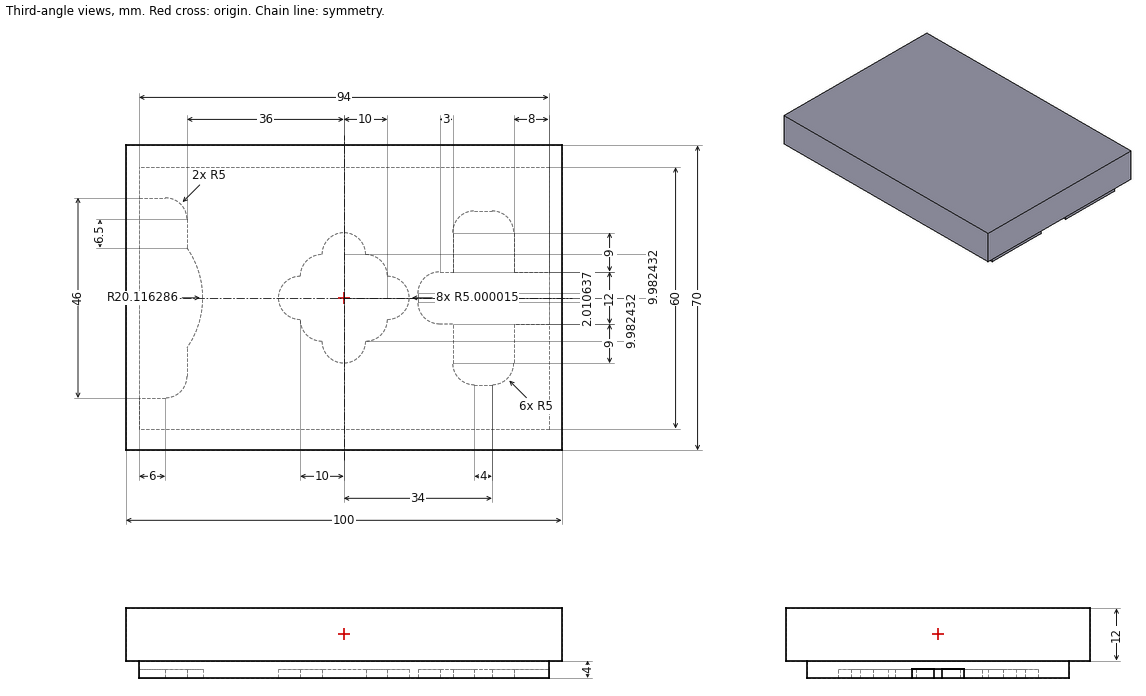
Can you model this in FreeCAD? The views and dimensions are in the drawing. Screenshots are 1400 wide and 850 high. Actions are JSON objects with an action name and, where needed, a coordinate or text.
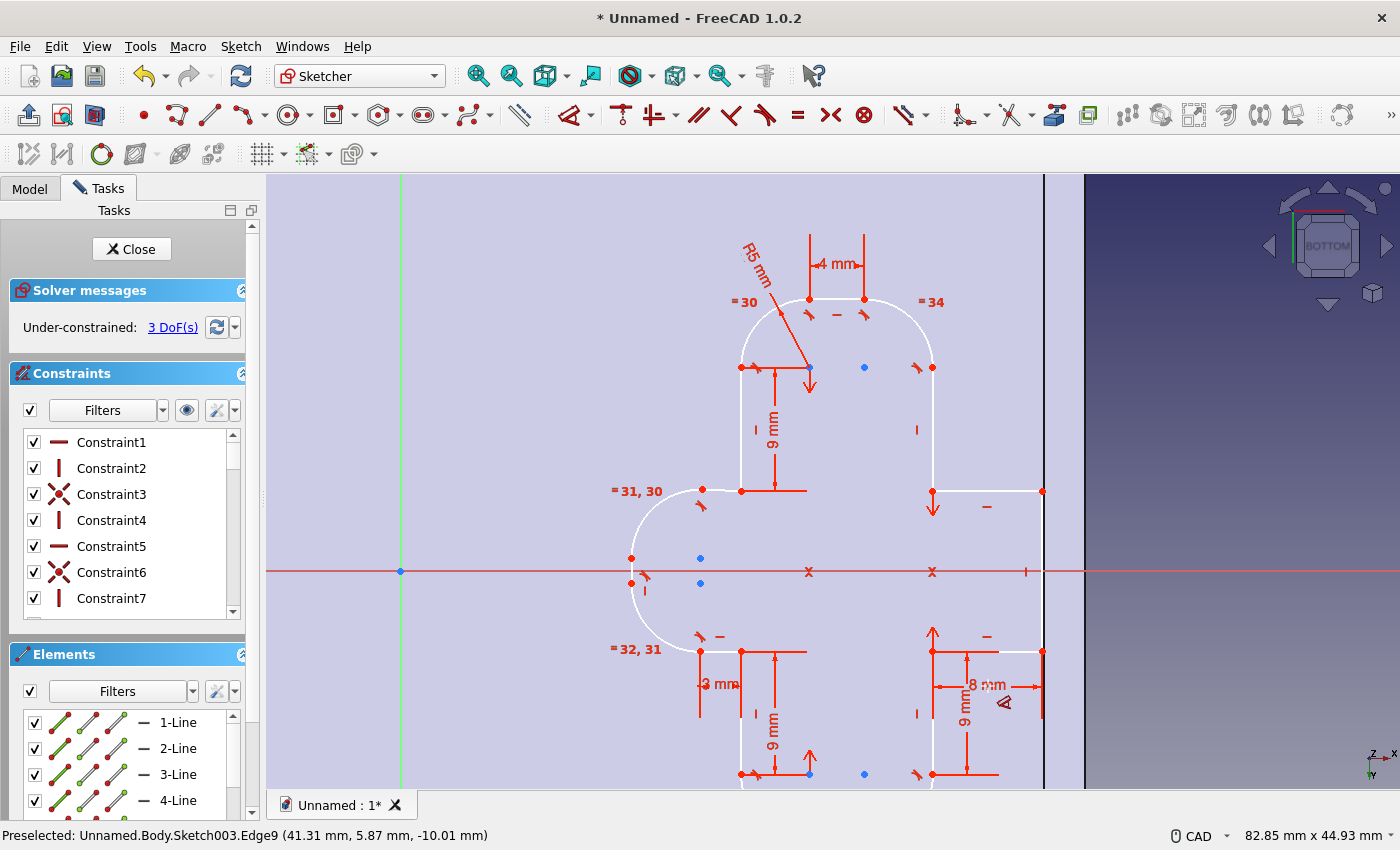
{"action": "left_click", "coordinate": [1042, 604]}
{"action": "left_click", "coordinate": [1076, 534]}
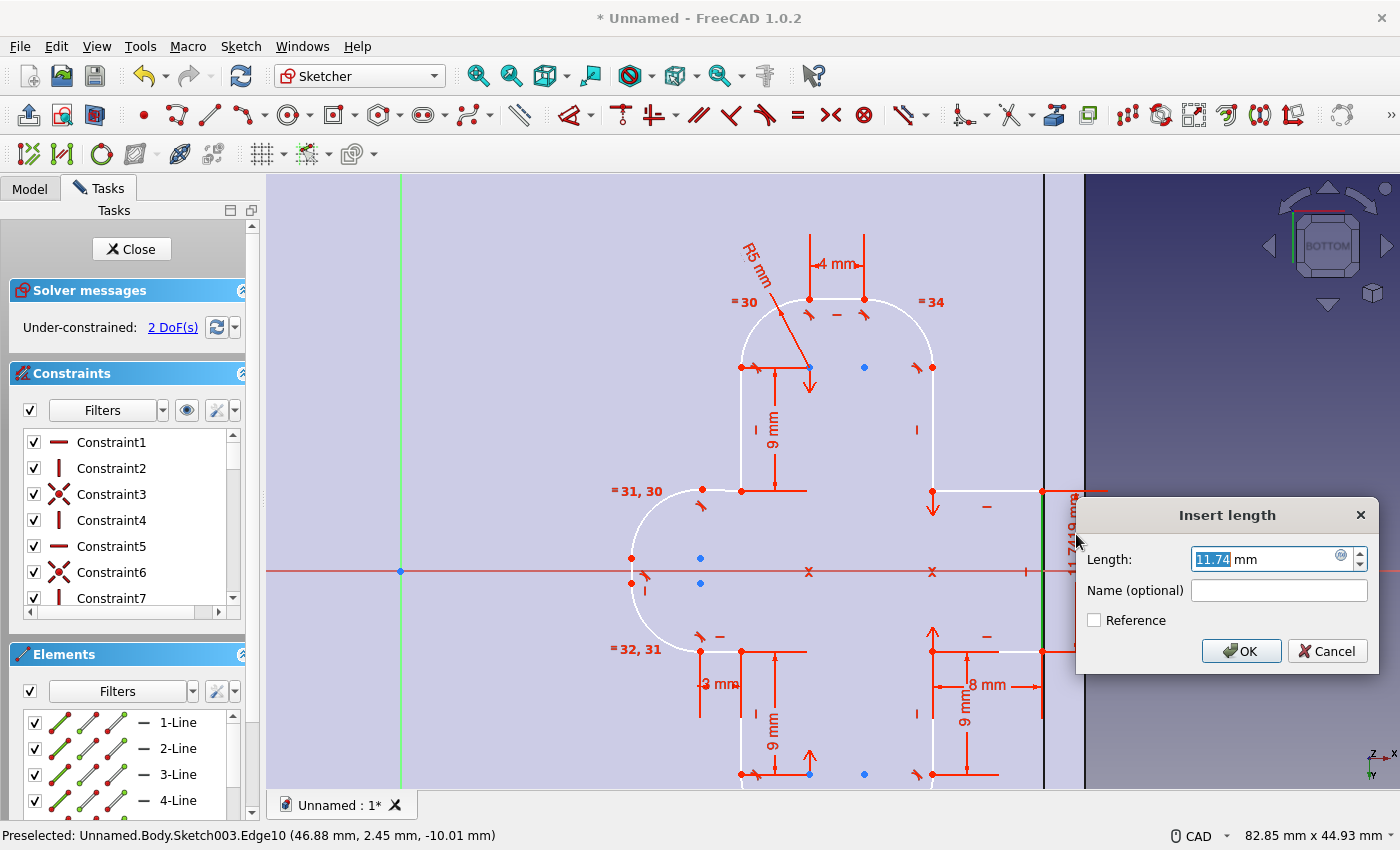
{"action": "type", "text": "12"}
{"action": "key", "text": "Return"}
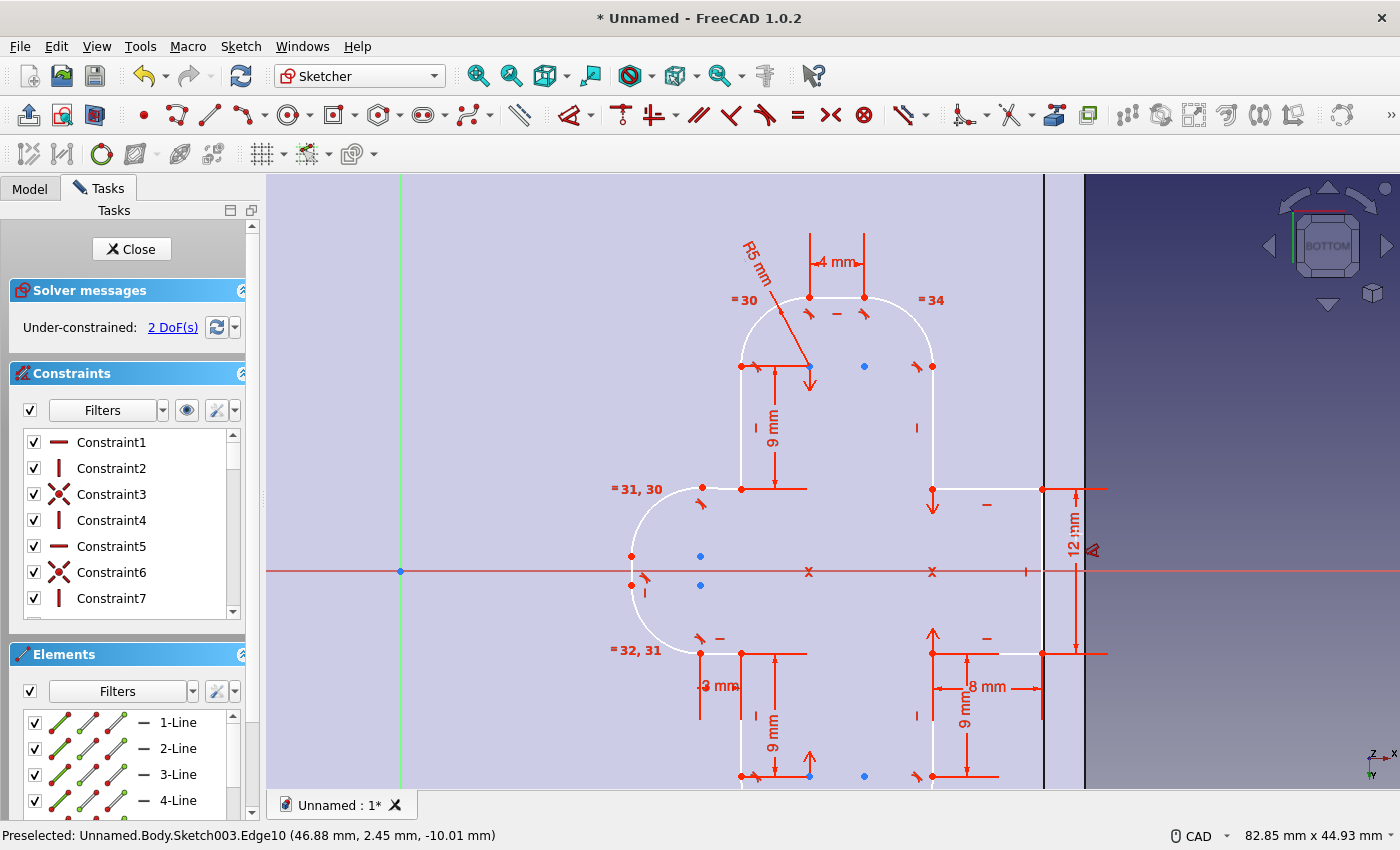
{"action": "left_click", "coordinate": [864, 298]}
{"action": "left_click", "coordinate": [633, 264]}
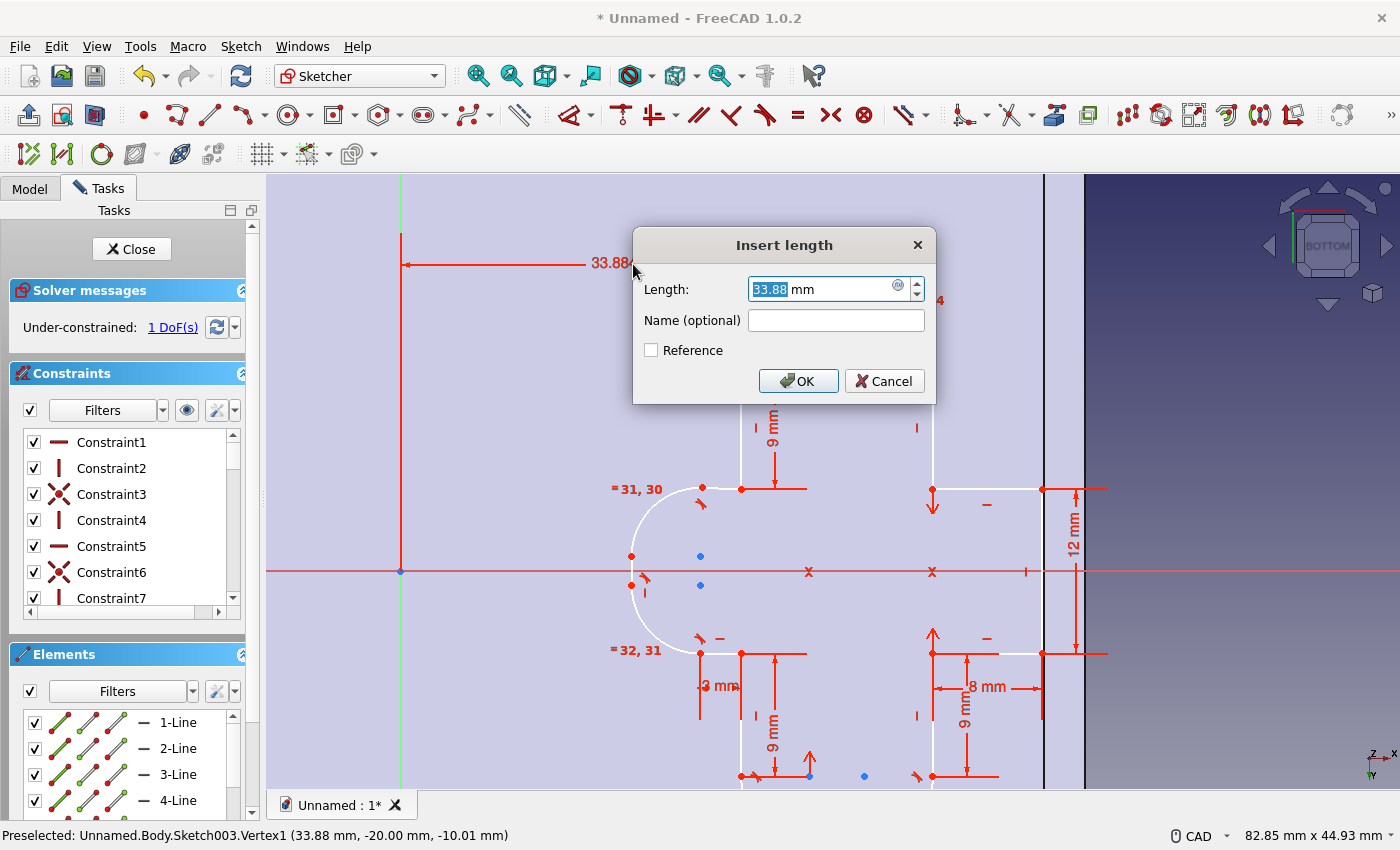
{"action": "type", "text": "34"}
{"action": "key", "text": "Return"}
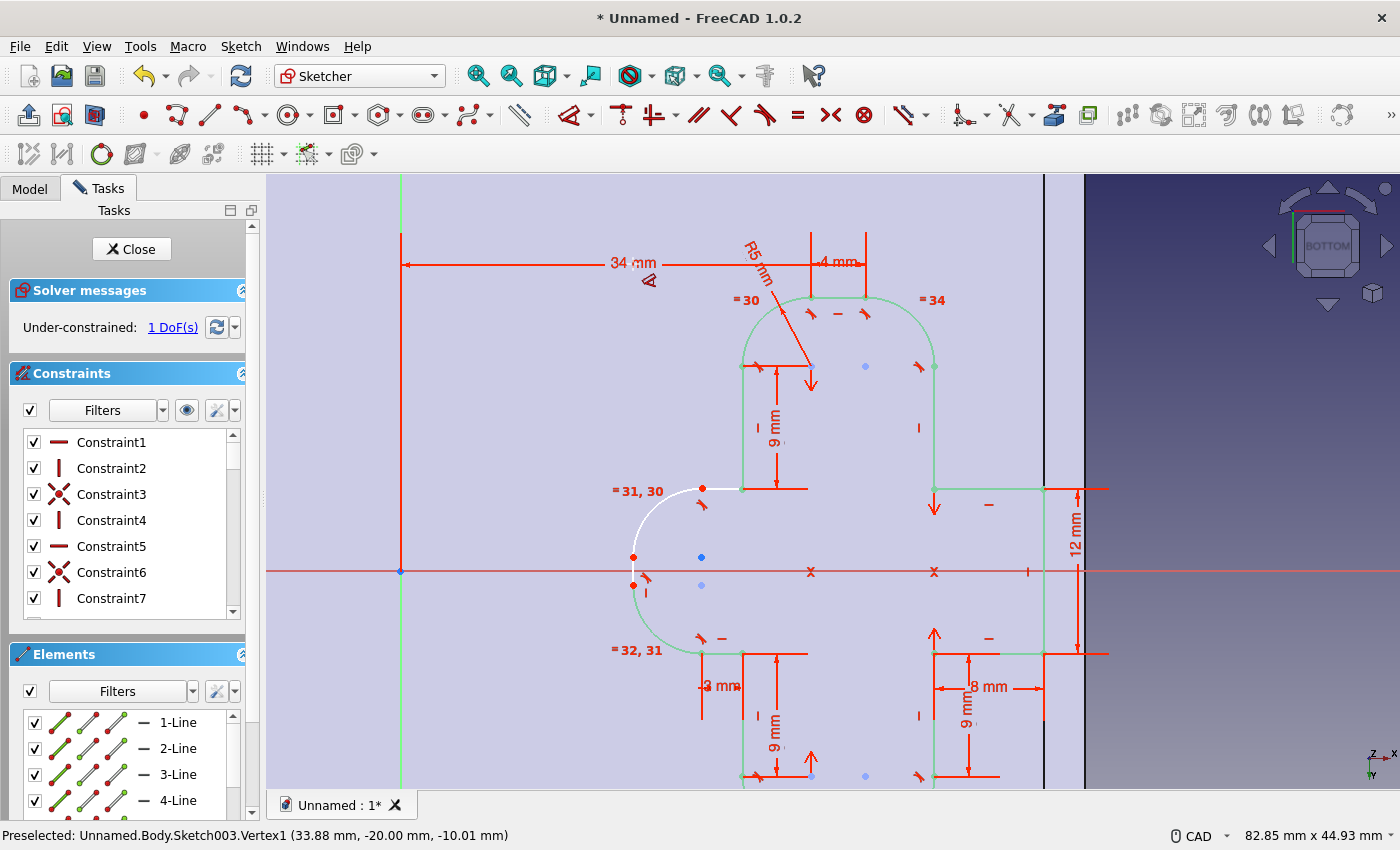
{"action": "scroll", "coordinate": [633, 568], "scroll_direction": "up", "scroll_amount": 2}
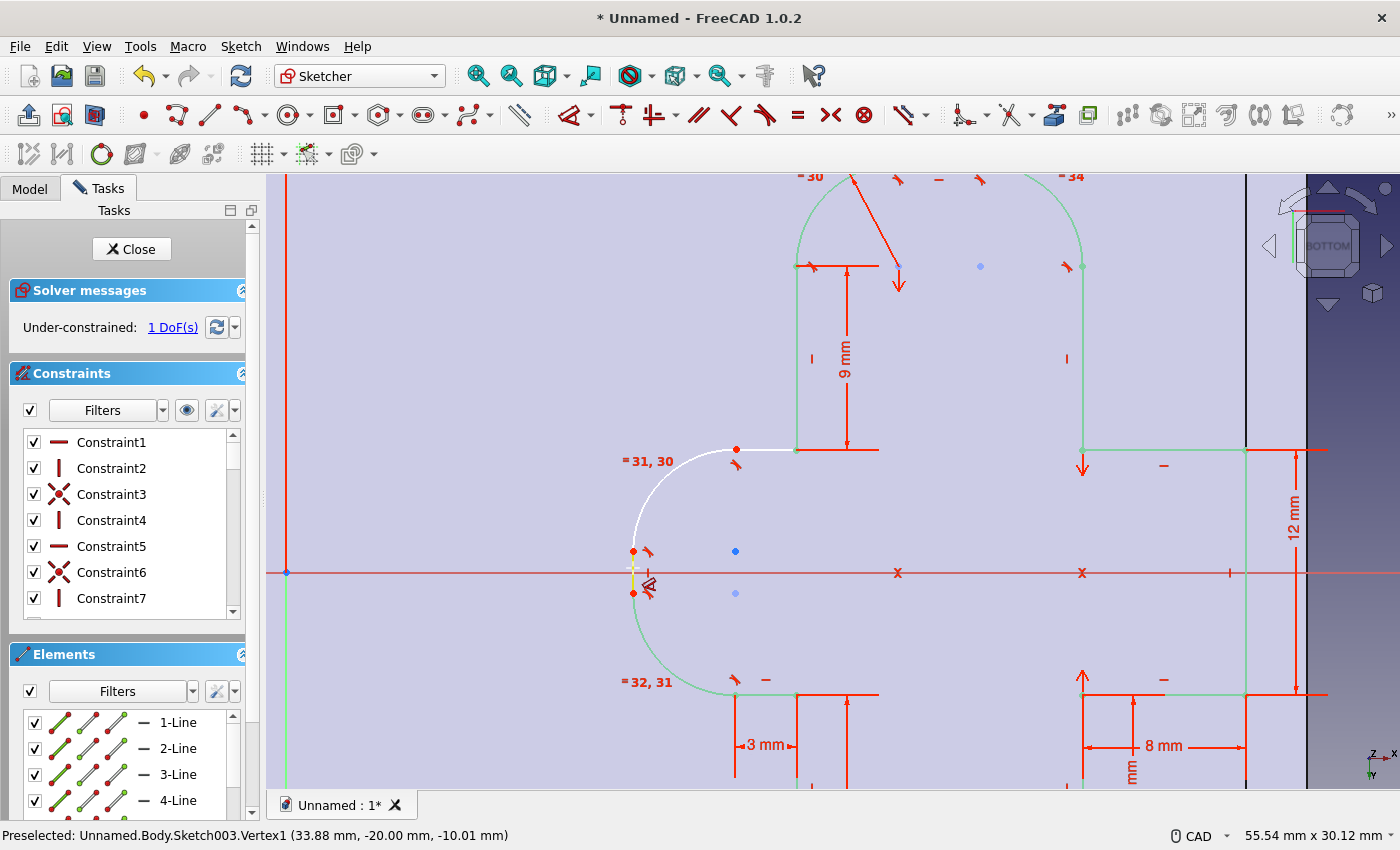
{"action": "left_click", "coordinate": [633, 568]}
{"action": "left_click", "coordinate": [599, 558]}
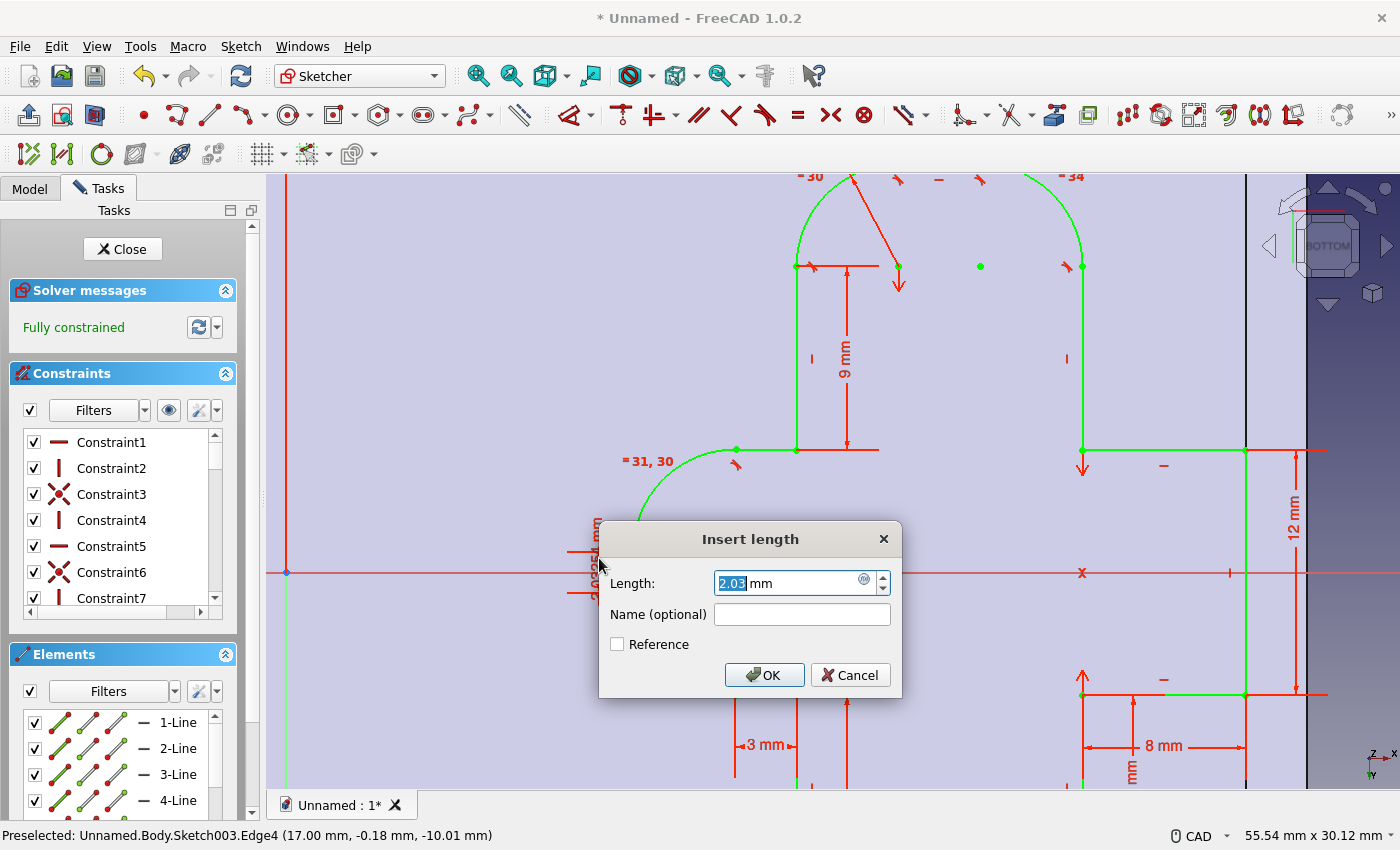
{"action": "type", "text": "2.010637"}
{"action": "key", "text": "Return"}
{"action": "key", "text": "Escape"}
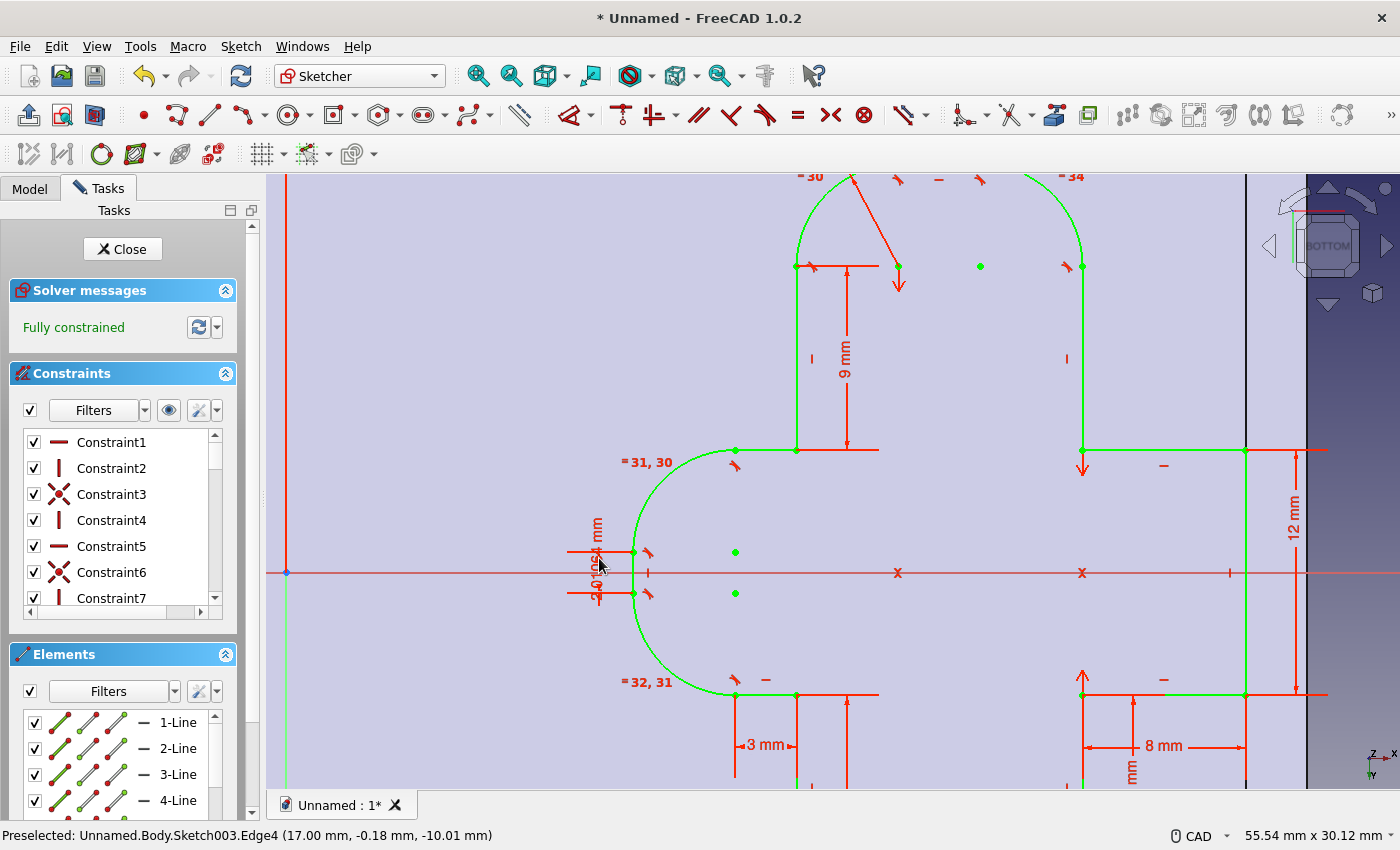
{"action": "left_click", "coordinate": [123, 249]}